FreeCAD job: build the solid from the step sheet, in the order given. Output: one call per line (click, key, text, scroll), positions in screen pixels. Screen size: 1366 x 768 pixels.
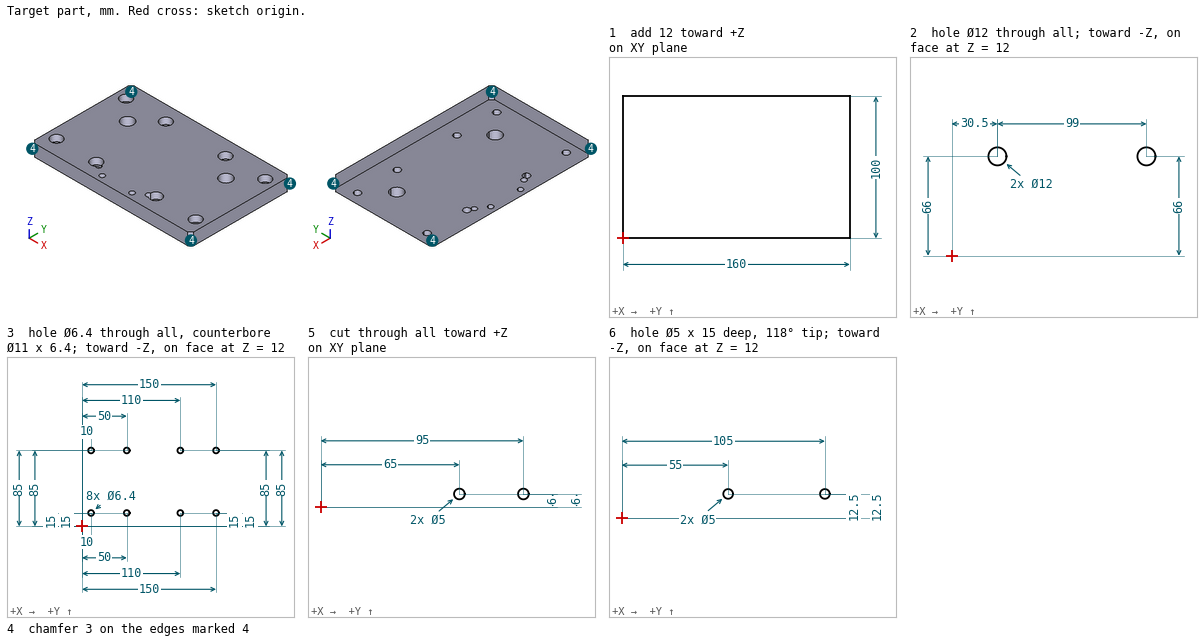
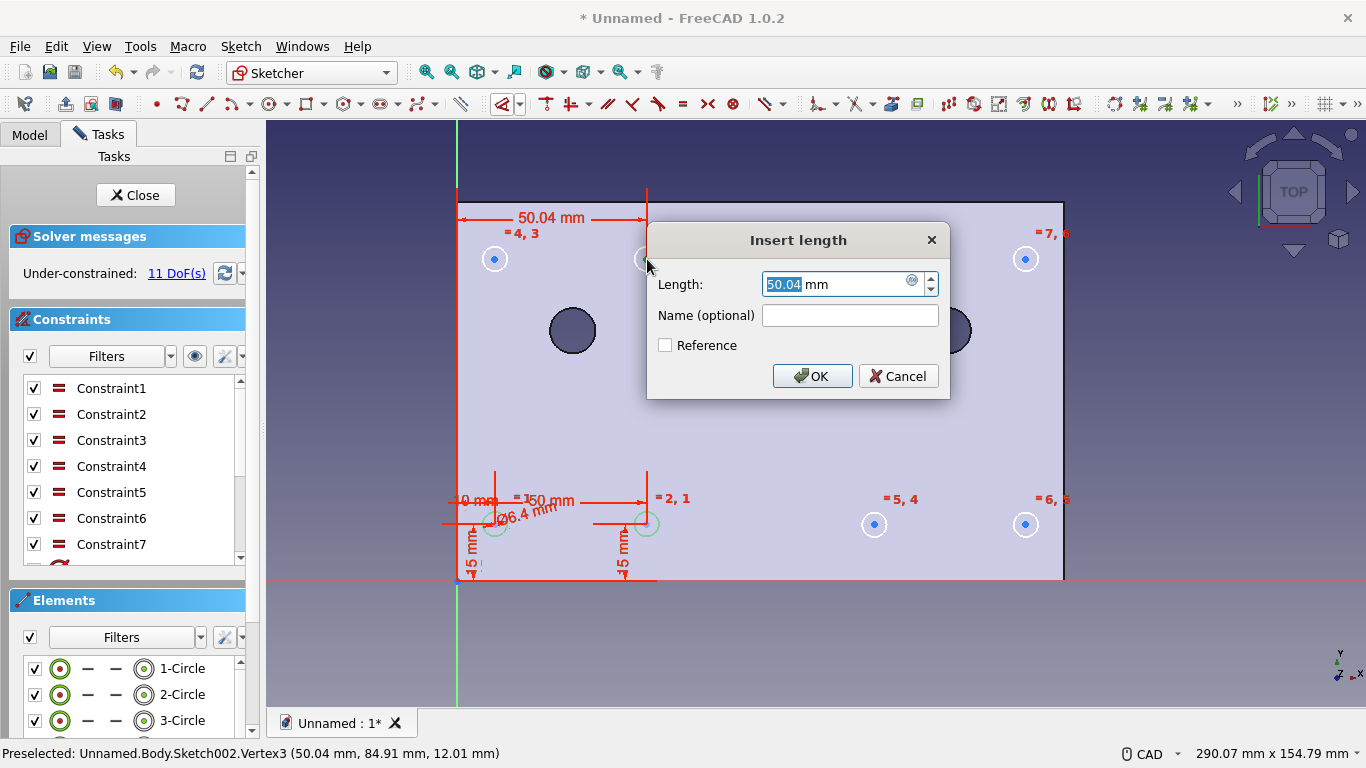
text(50)
key(Return)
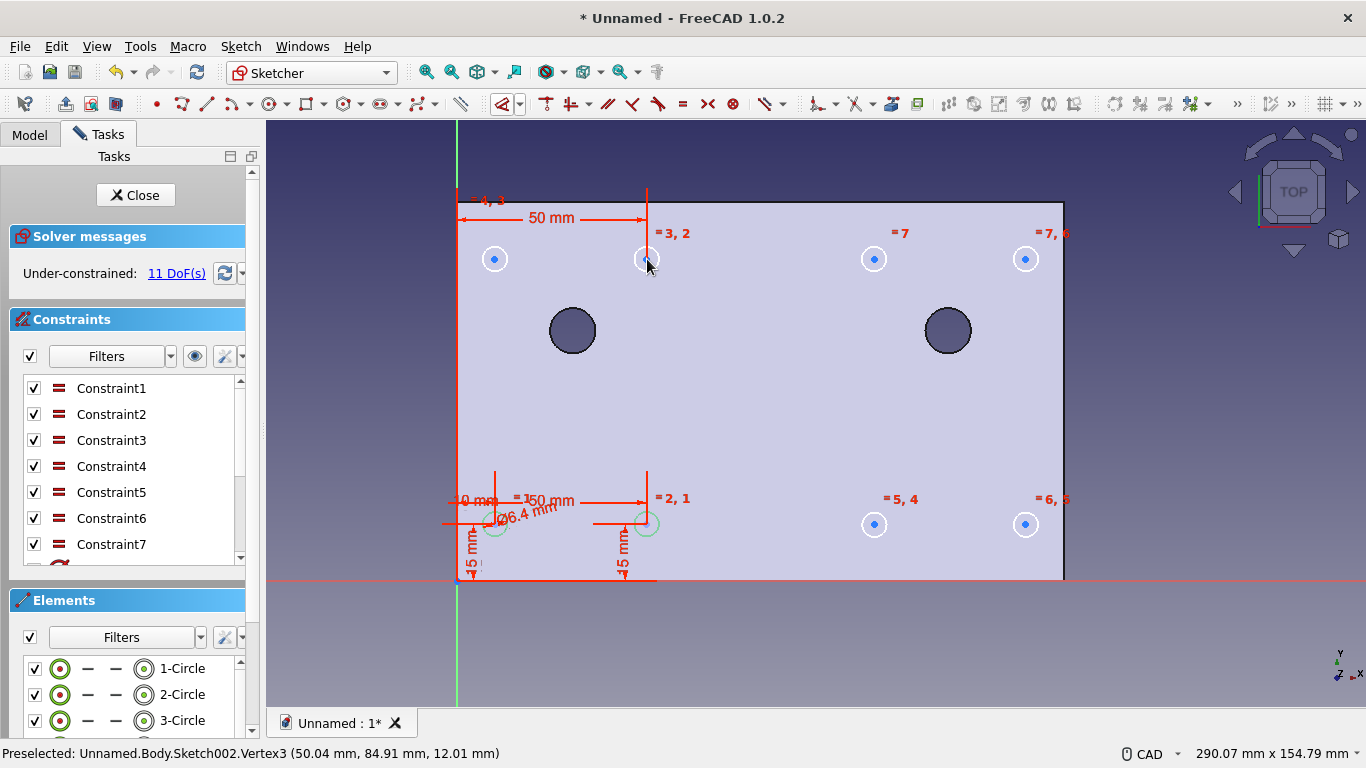
click(647, 259)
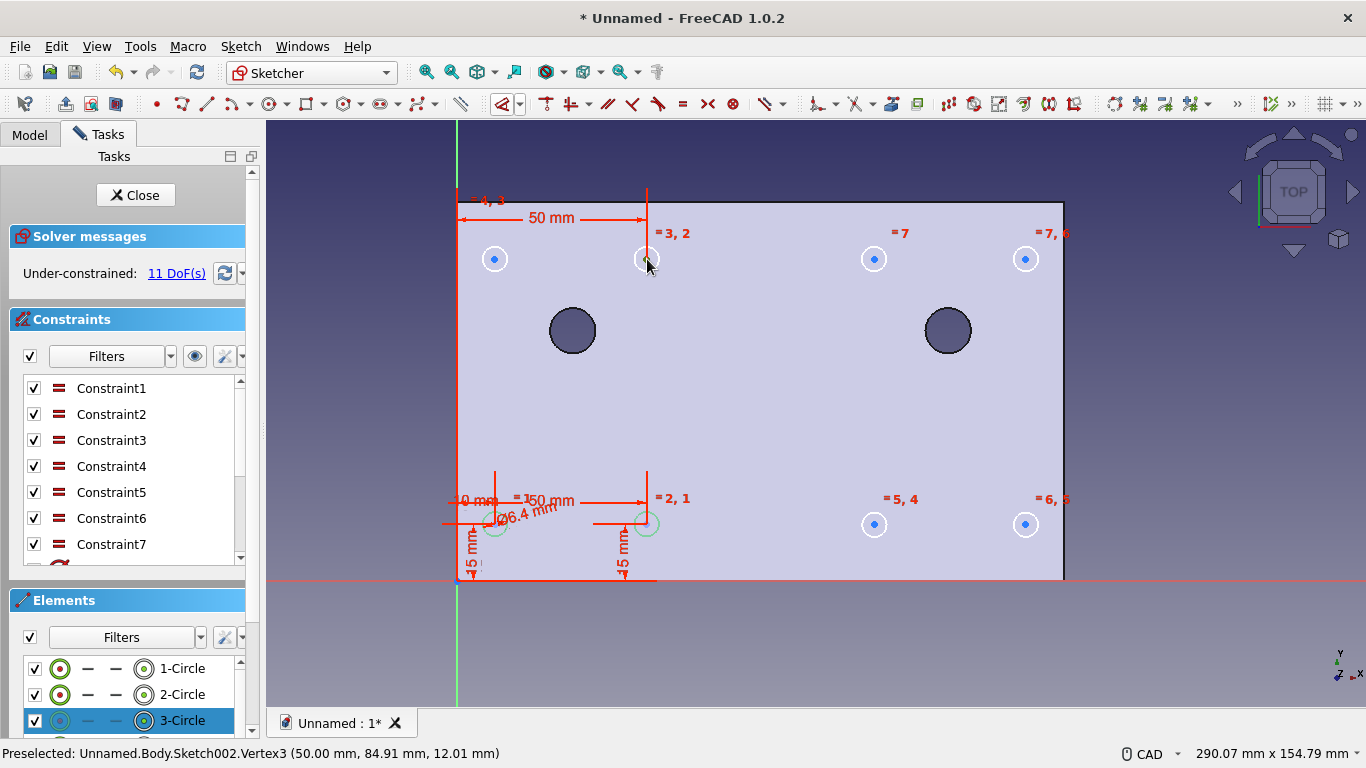
key(i)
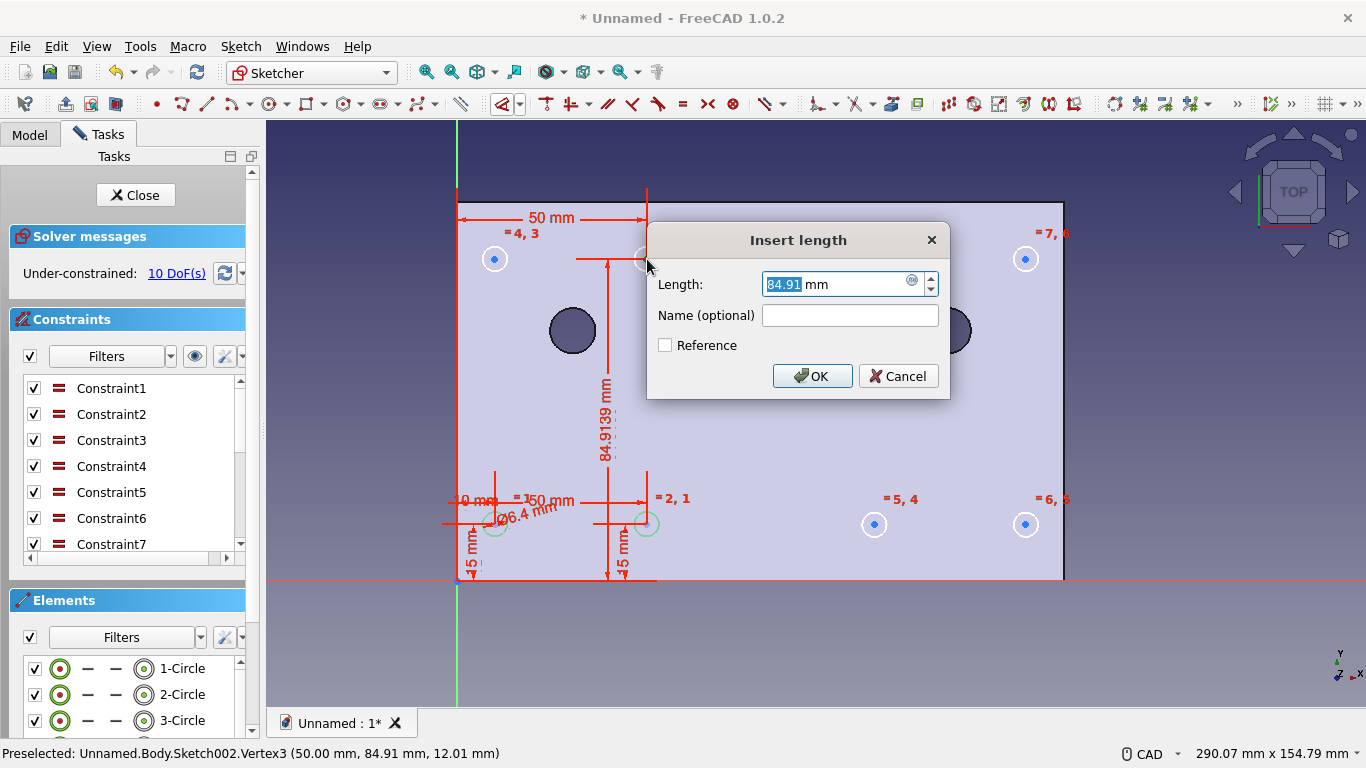
text(85)
key(Return)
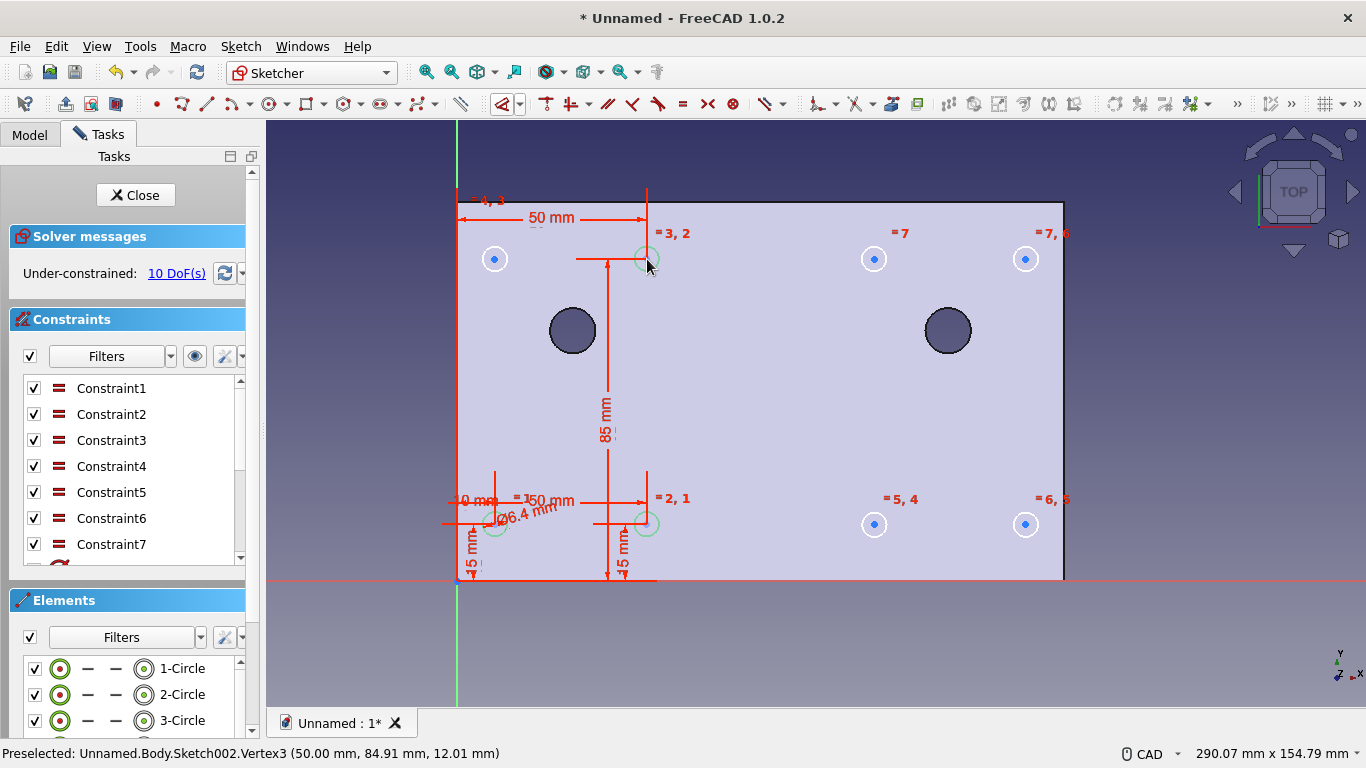
click(495, 259)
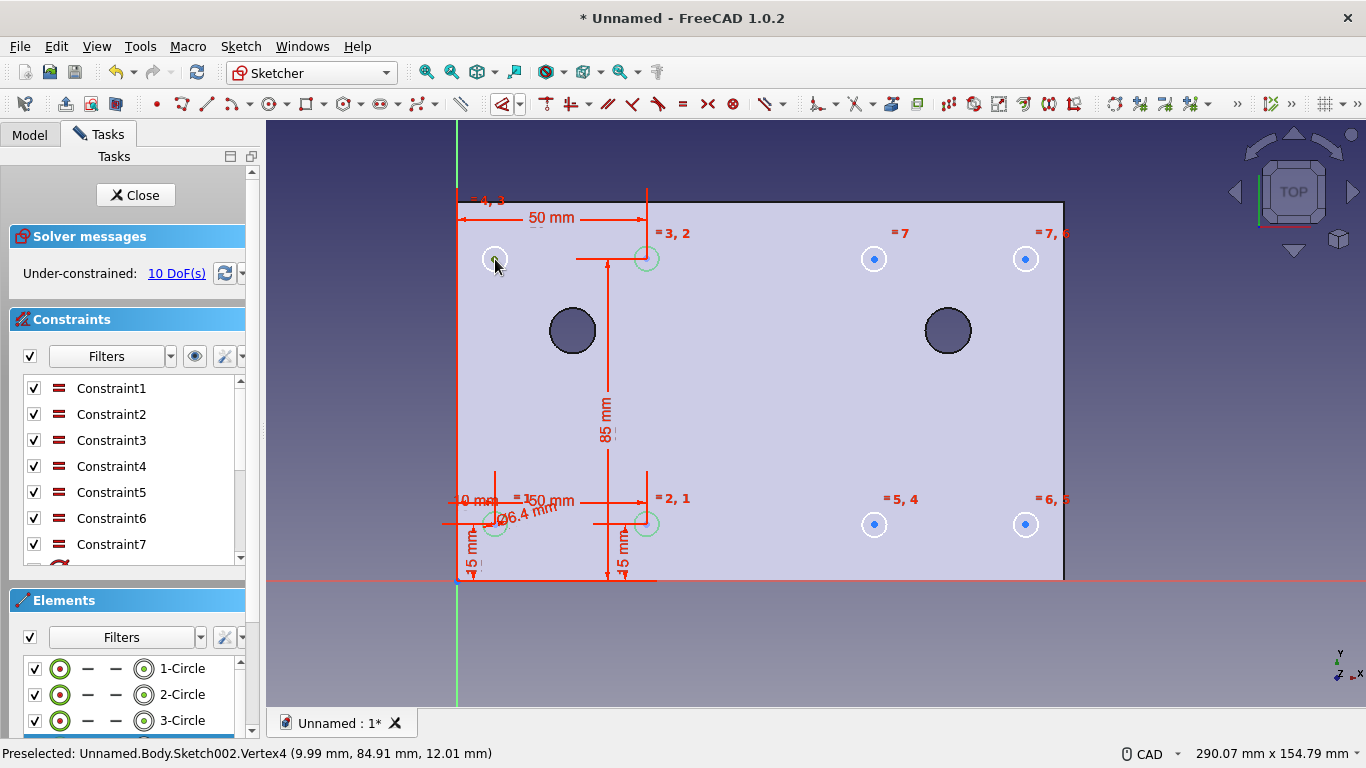
key(l)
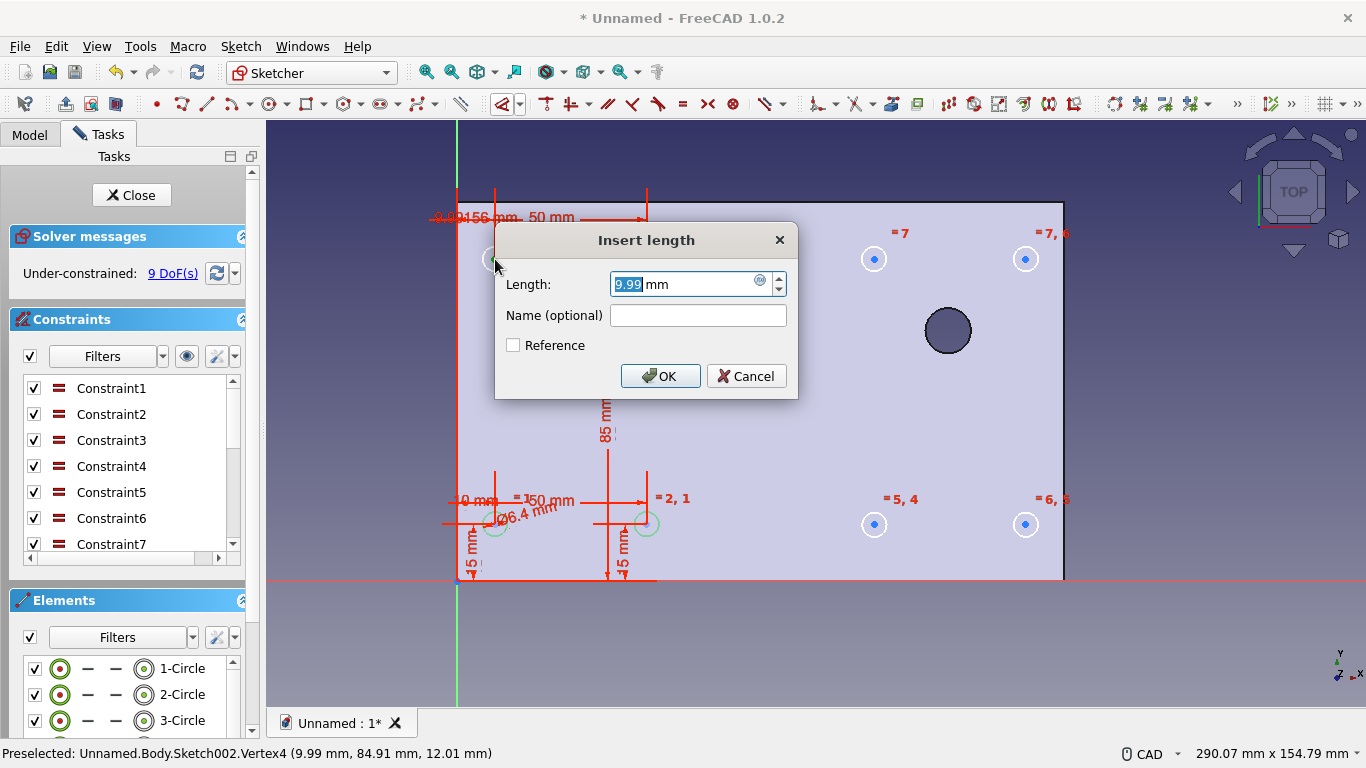
text(10)
key(Return)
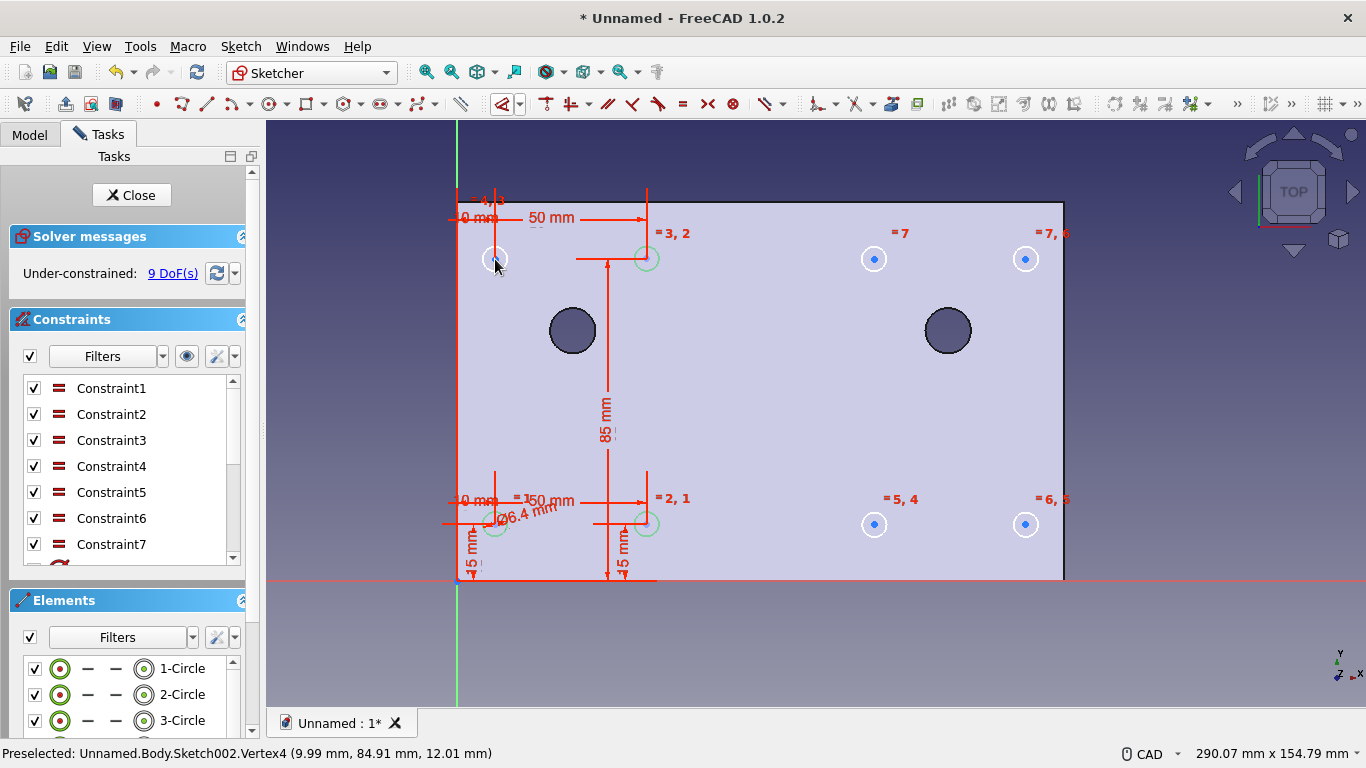
click(495, 259)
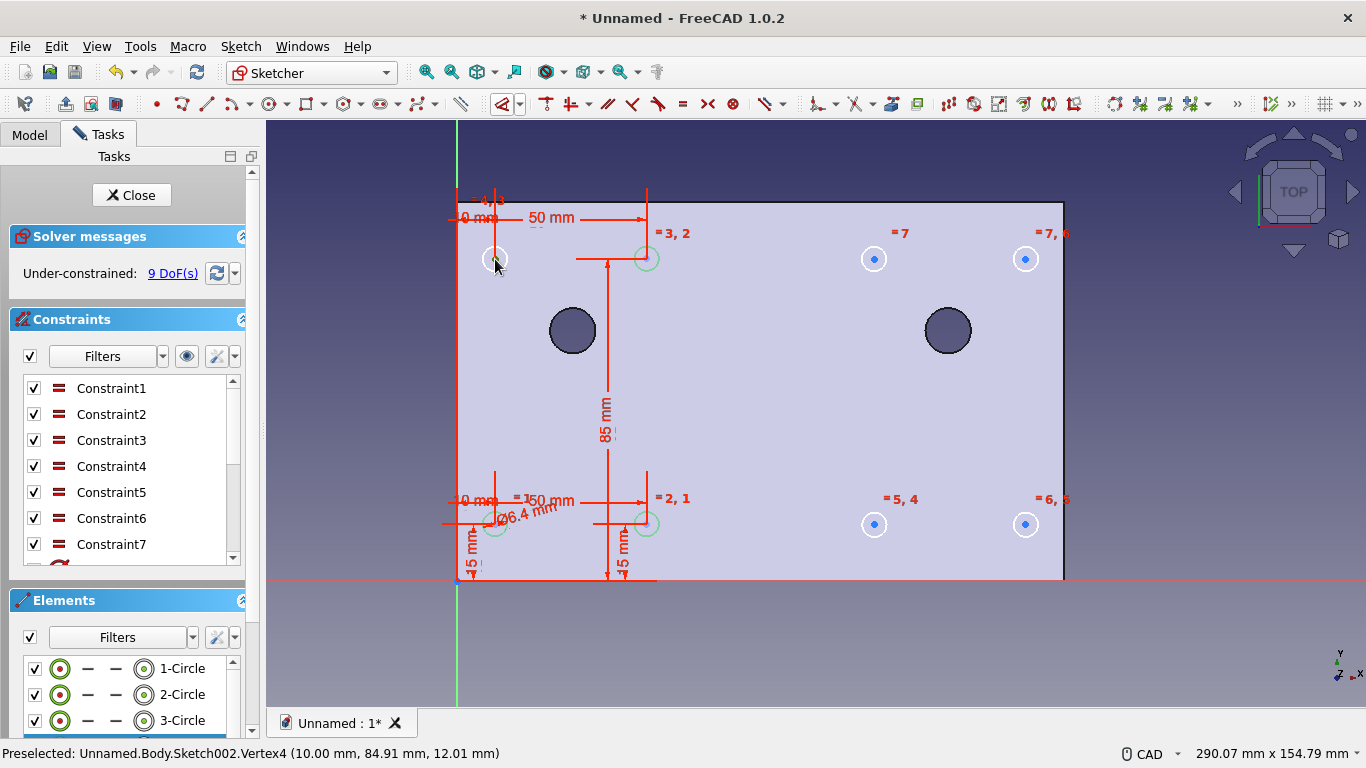
key(i)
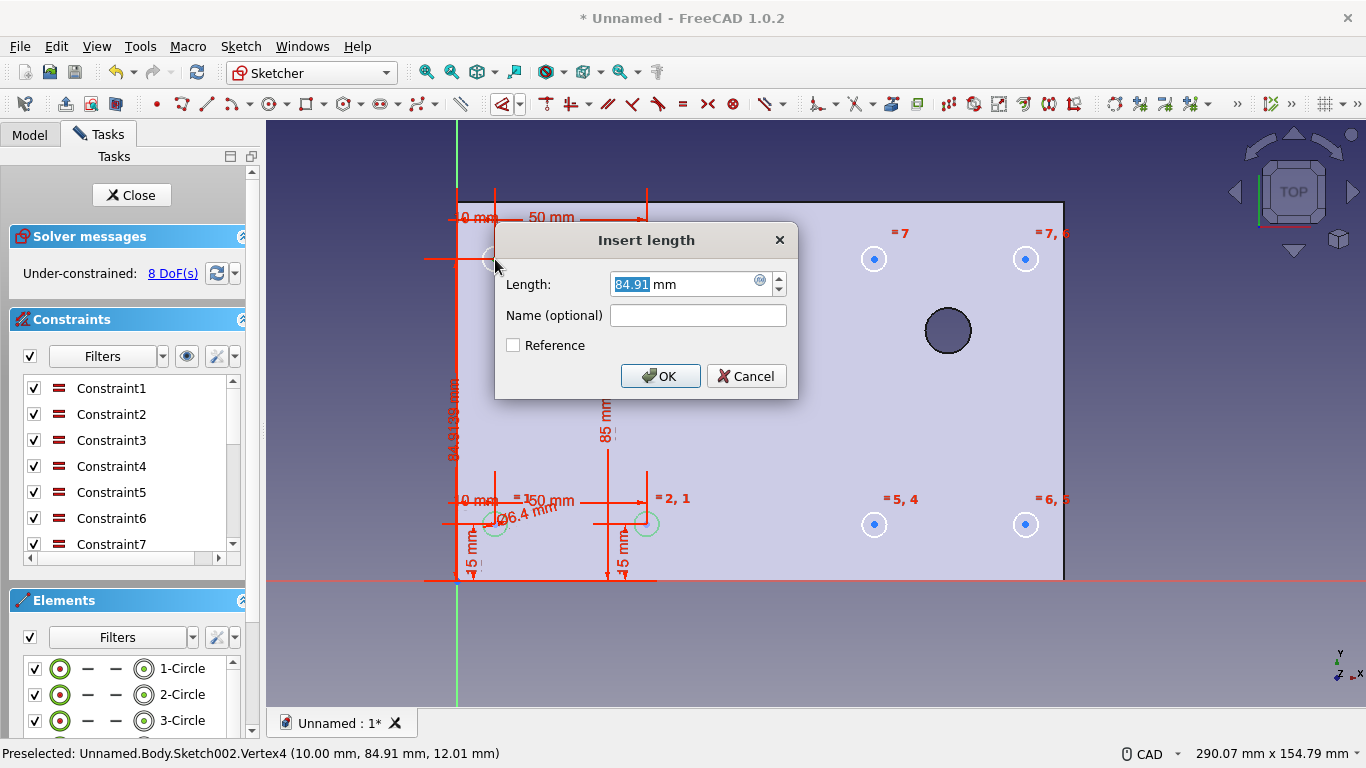
text(85)
key(Return)